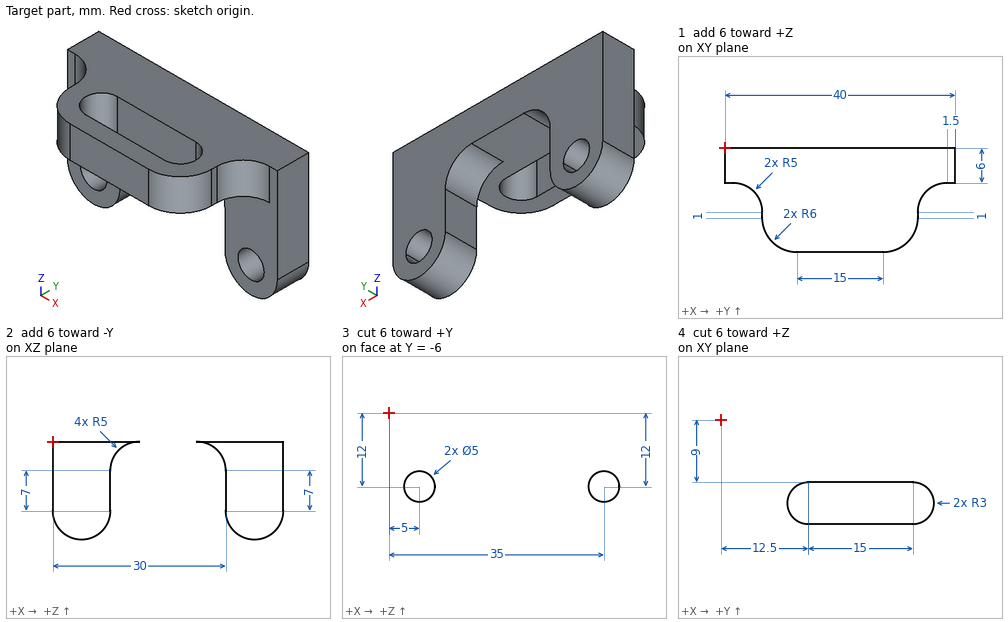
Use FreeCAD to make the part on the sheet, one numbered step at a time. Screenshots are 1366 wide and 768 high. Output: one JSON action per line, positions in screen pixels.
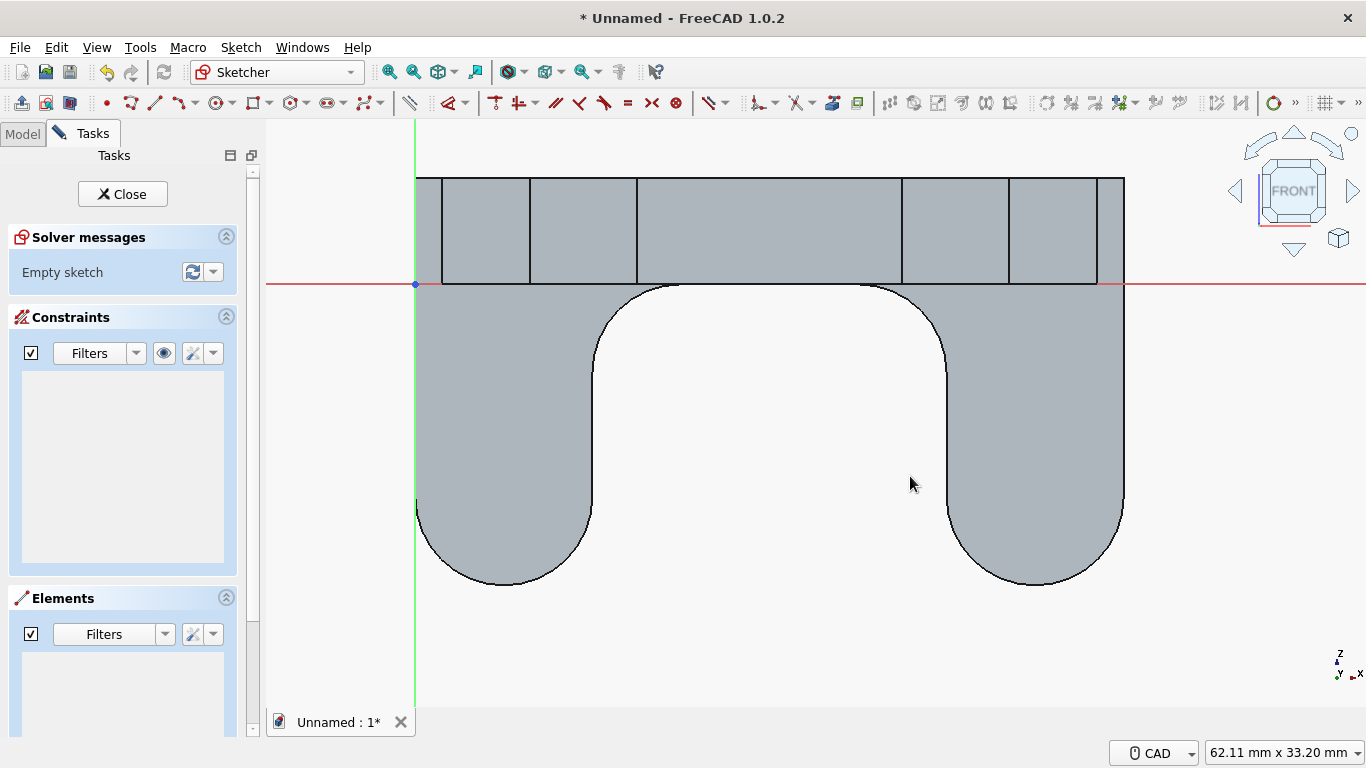
{"action": "left_click", "coordinate": [216, 104]}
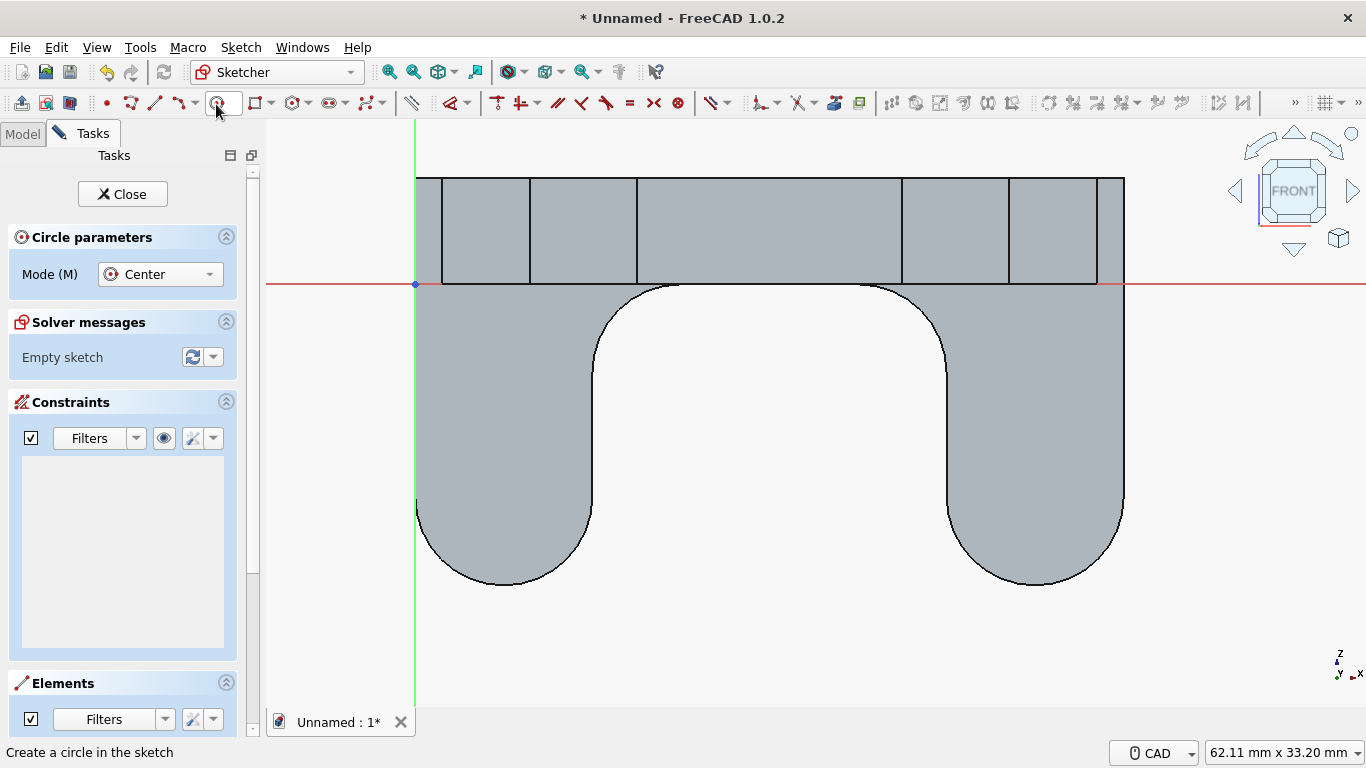
{"action": "left_click", "coordinate": [504, 497]}
{"action": "left_click", "coordinate": [535, 466]}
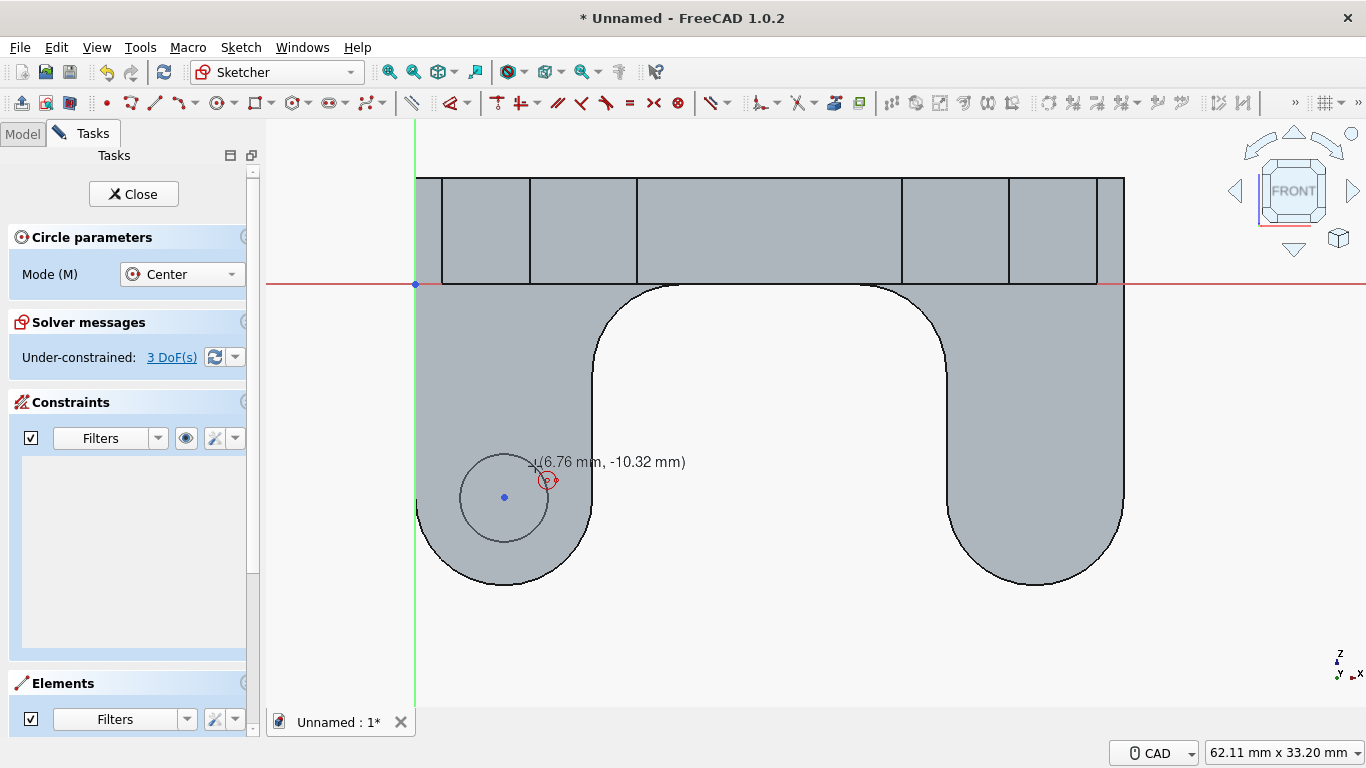
{"action": "left_click", "coordinate": [1035, 497]}
{"action": "left_click", "coordinate": [1066, 466]}
{"action": "key", "text": "Escape"}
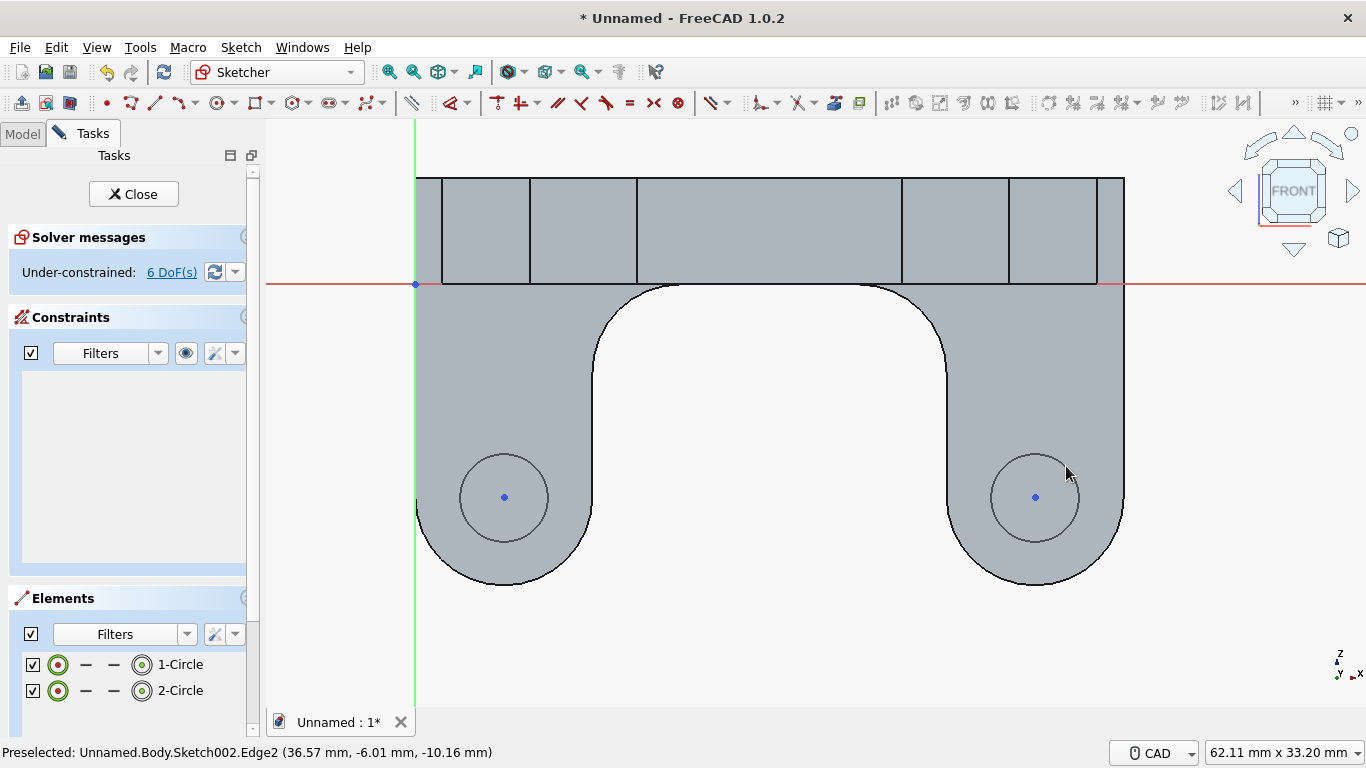
{"action": "left_click", "coordinate": [535, 467]}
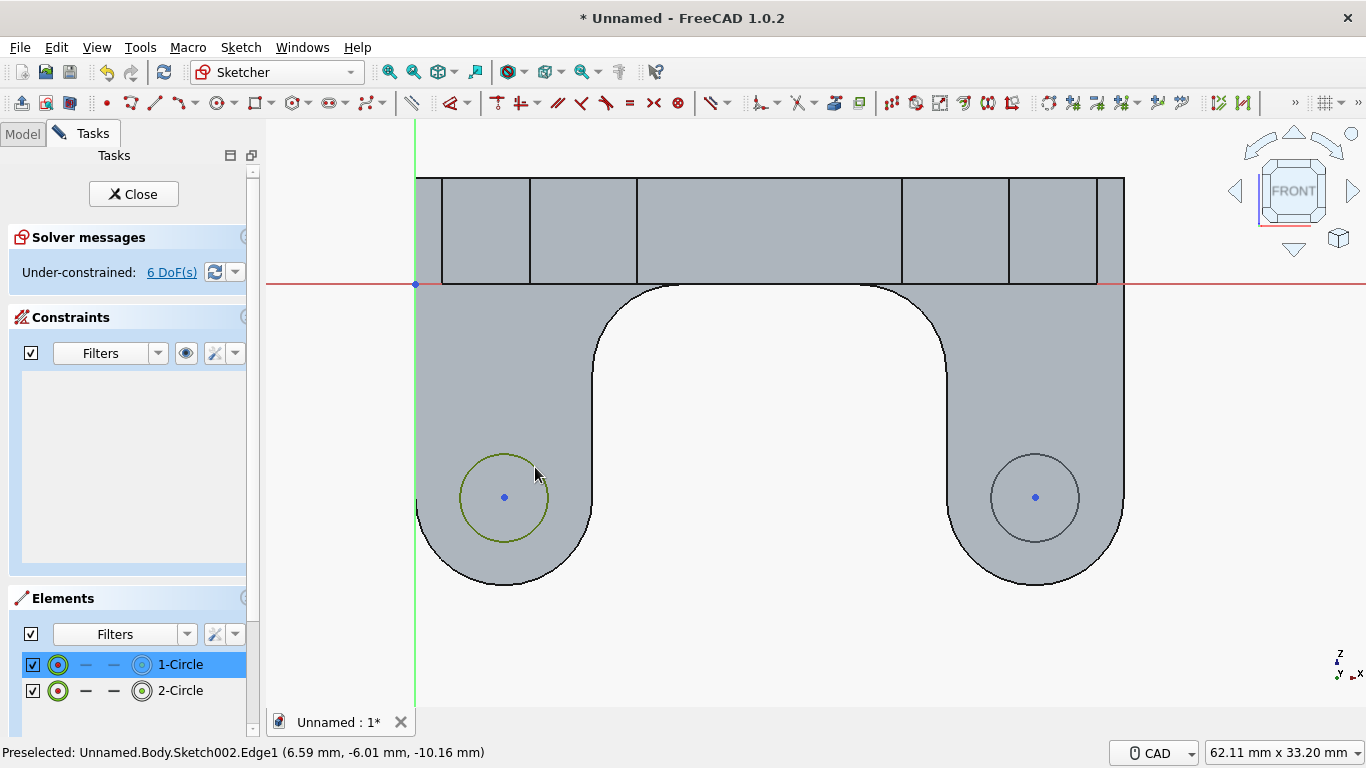
{"action": "left_click", "coordinate": [1066, 467]}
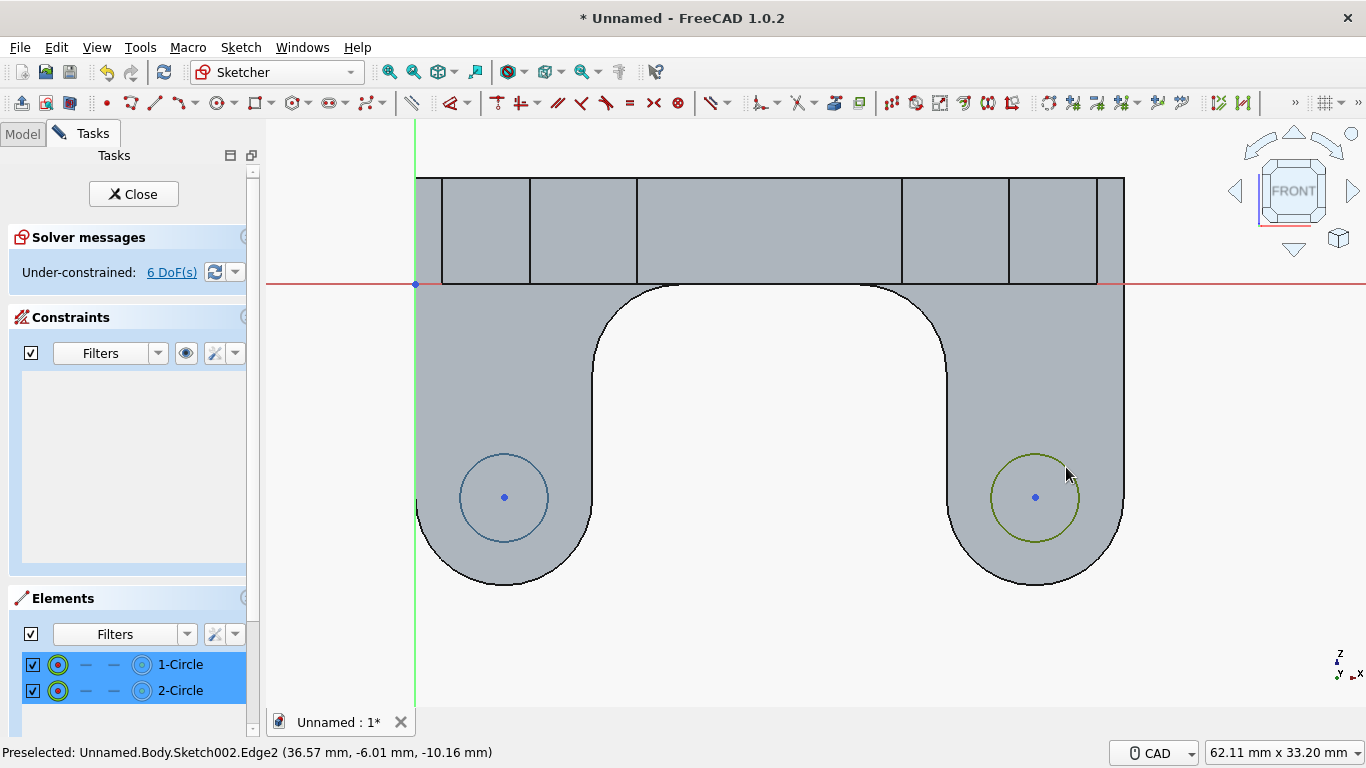
{"action": "left_click", "coordinate": [630, 104]}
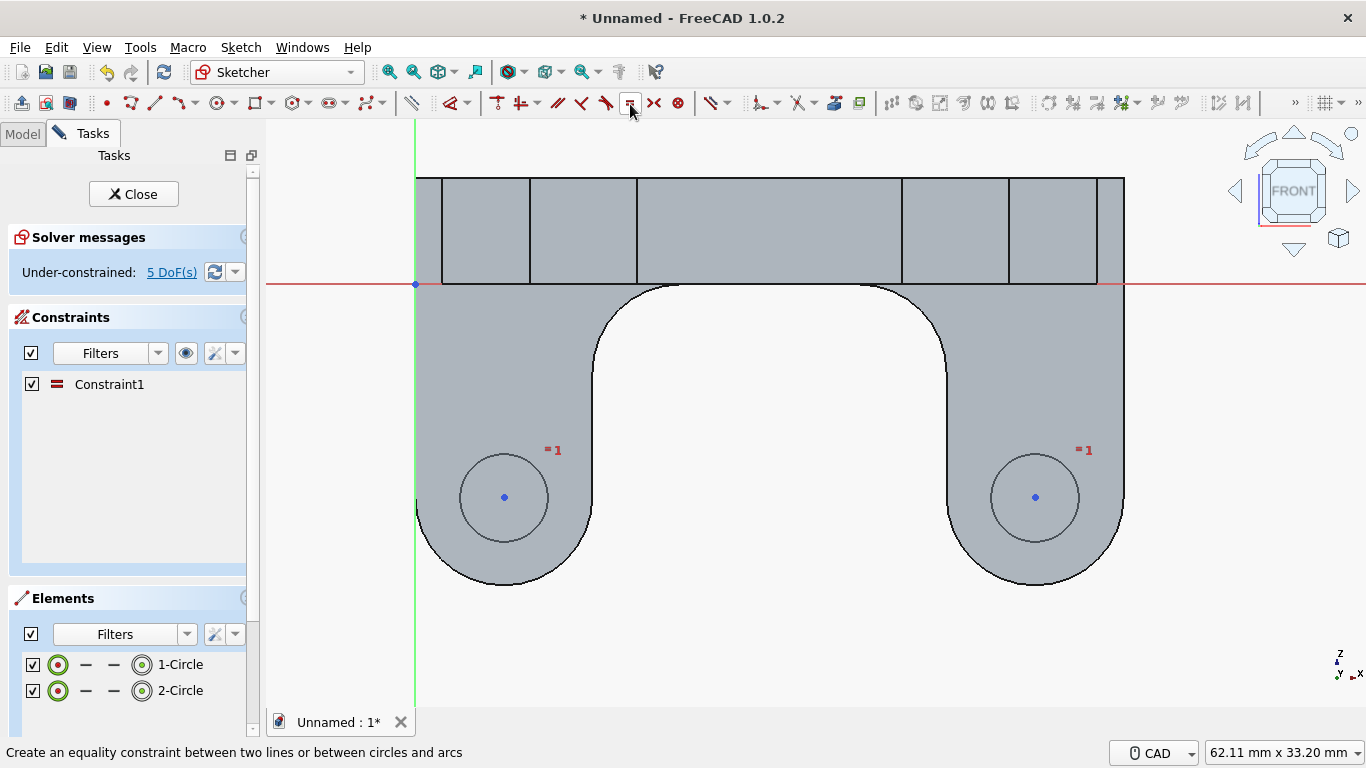
{"action": "left_click", "coordinate": [450, 104]}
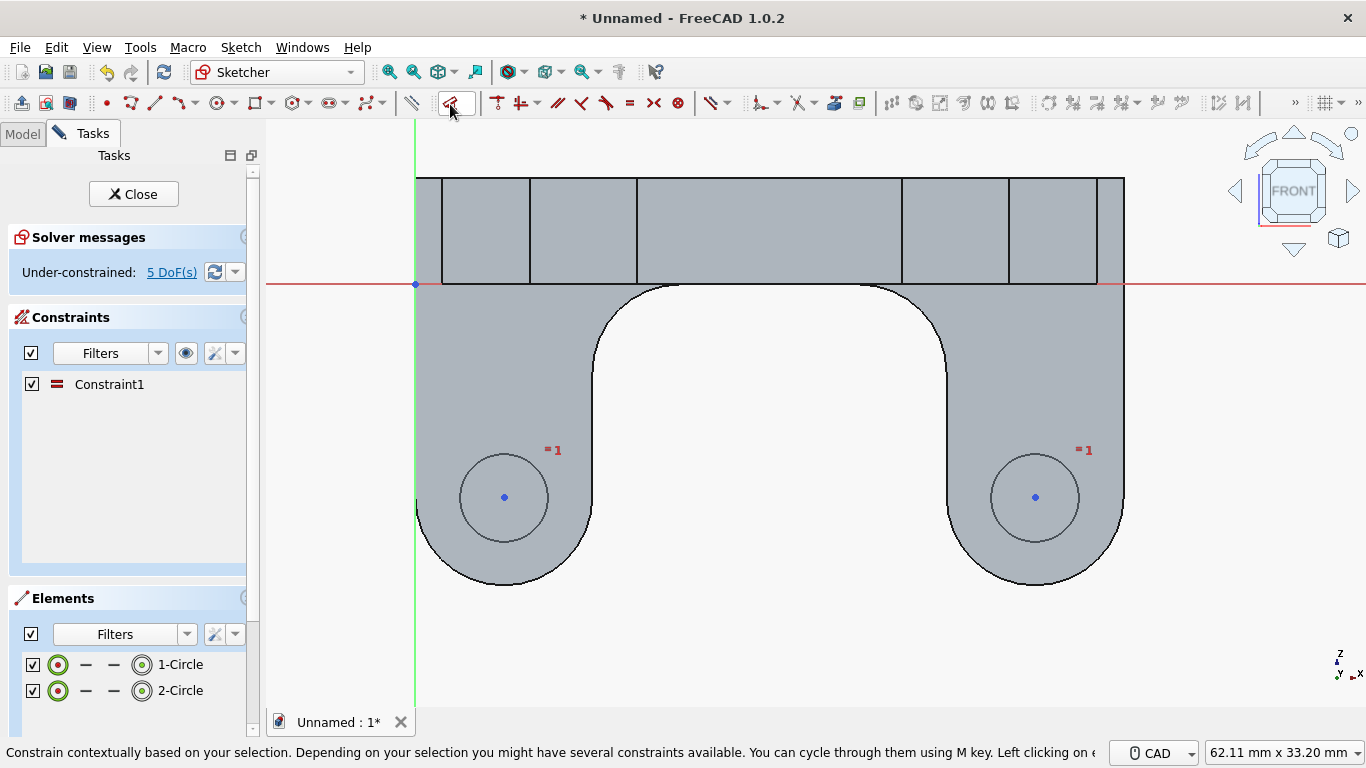
{"action": "left_click", "coordinate": [535, 467]}
{"action": "left_click", "coordinate": [558, 444]}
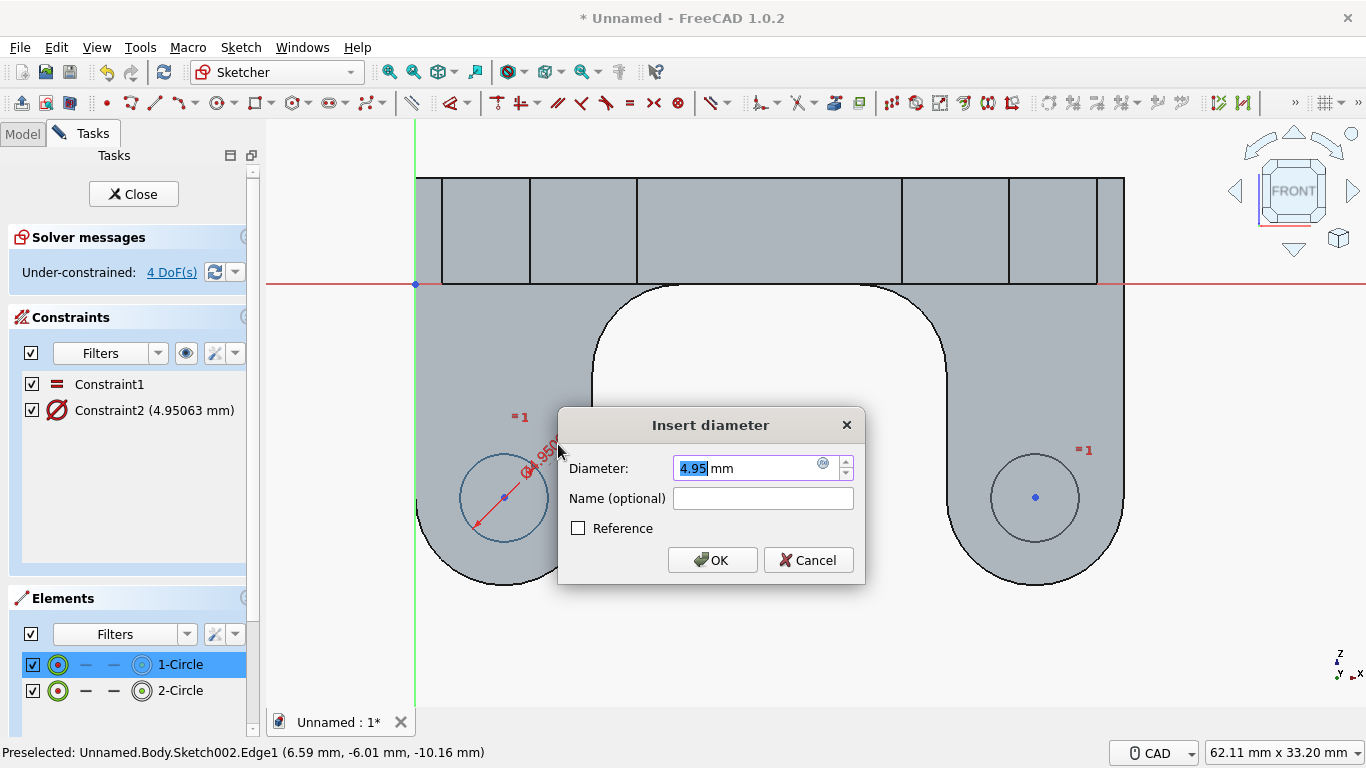
{"action": "type", "text": "5"}
{"action": "key", "text": "Return"}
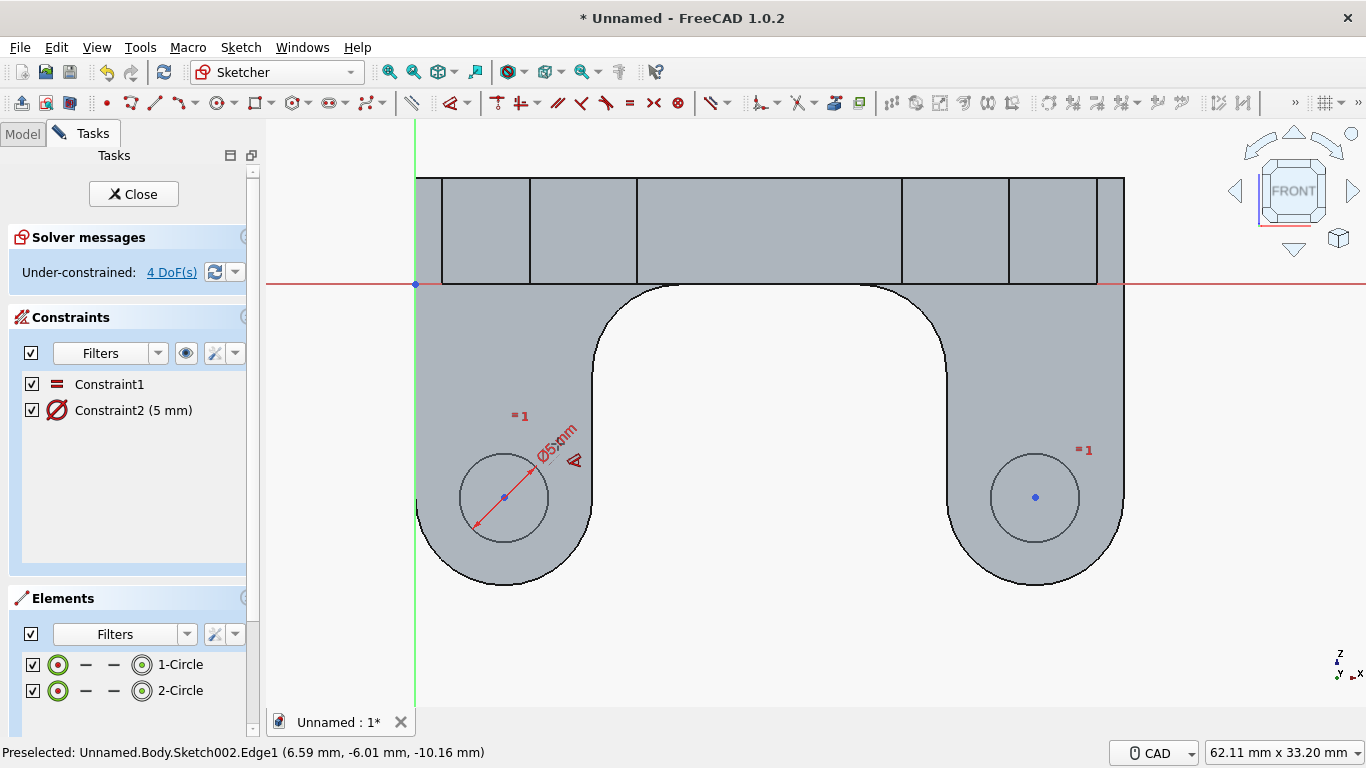
{"action": "left_click", "coordinate": [504, 498]}
{"action": "left_click", "coordinate": [460, 250]}